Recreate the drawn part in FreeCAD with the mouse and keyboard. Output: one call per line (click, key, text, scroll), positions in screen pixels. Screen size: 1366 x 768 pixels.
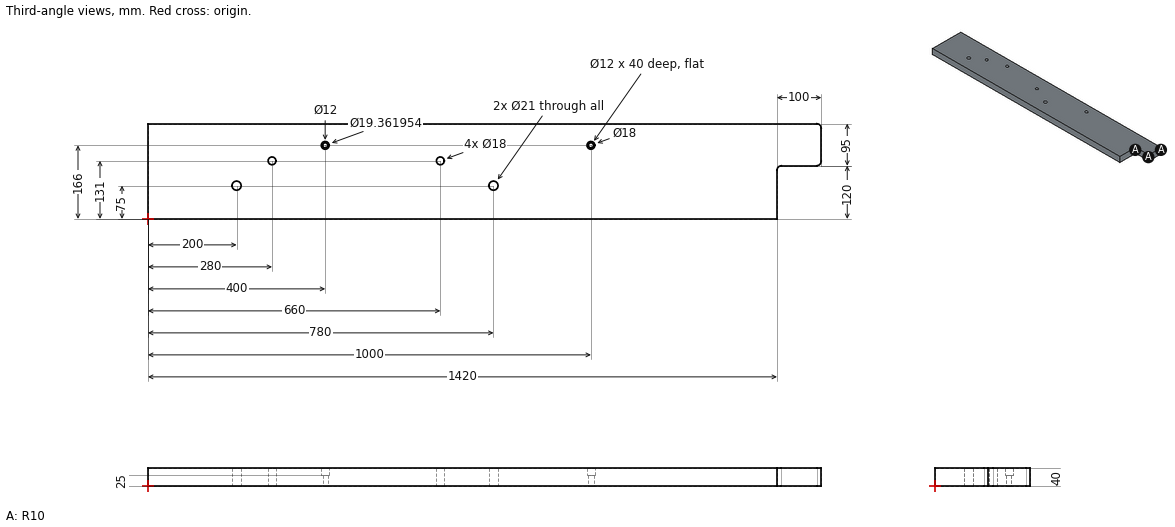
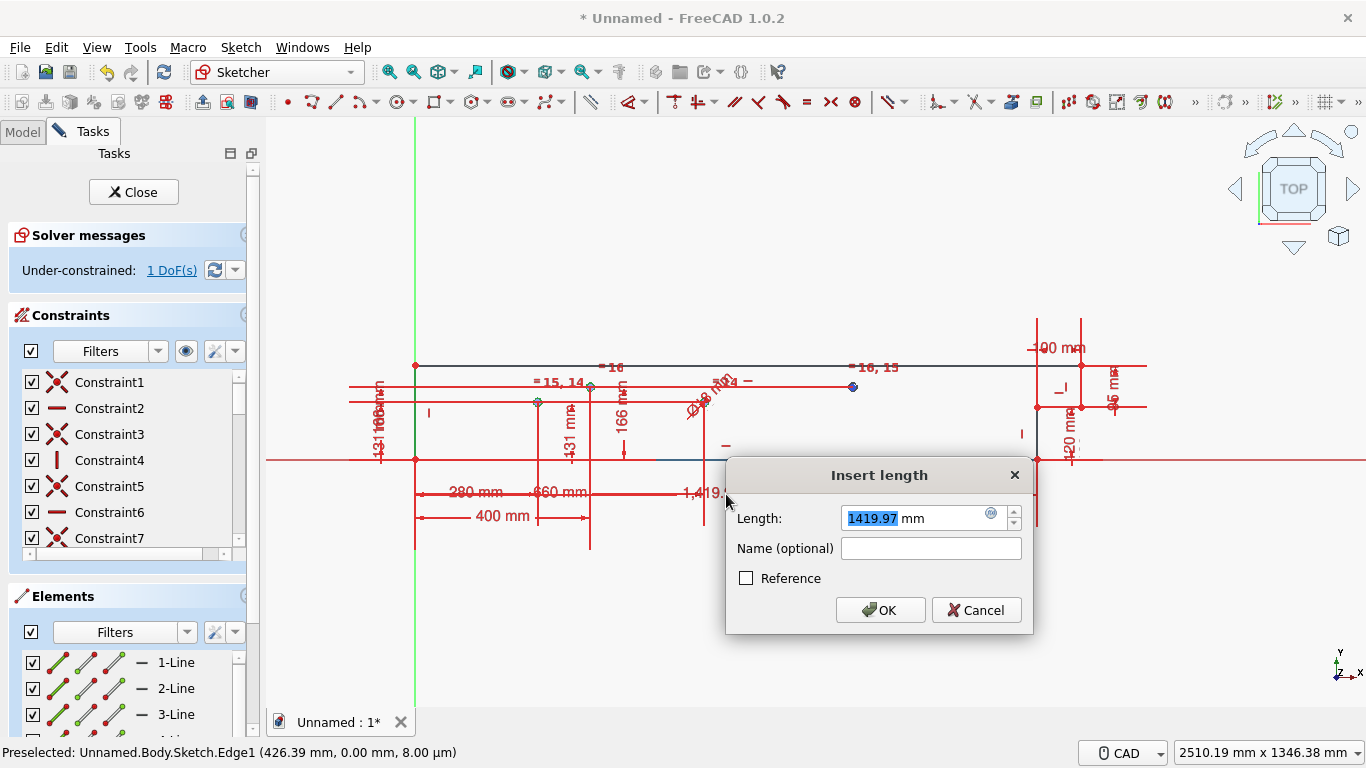
text(1420)
key(Return)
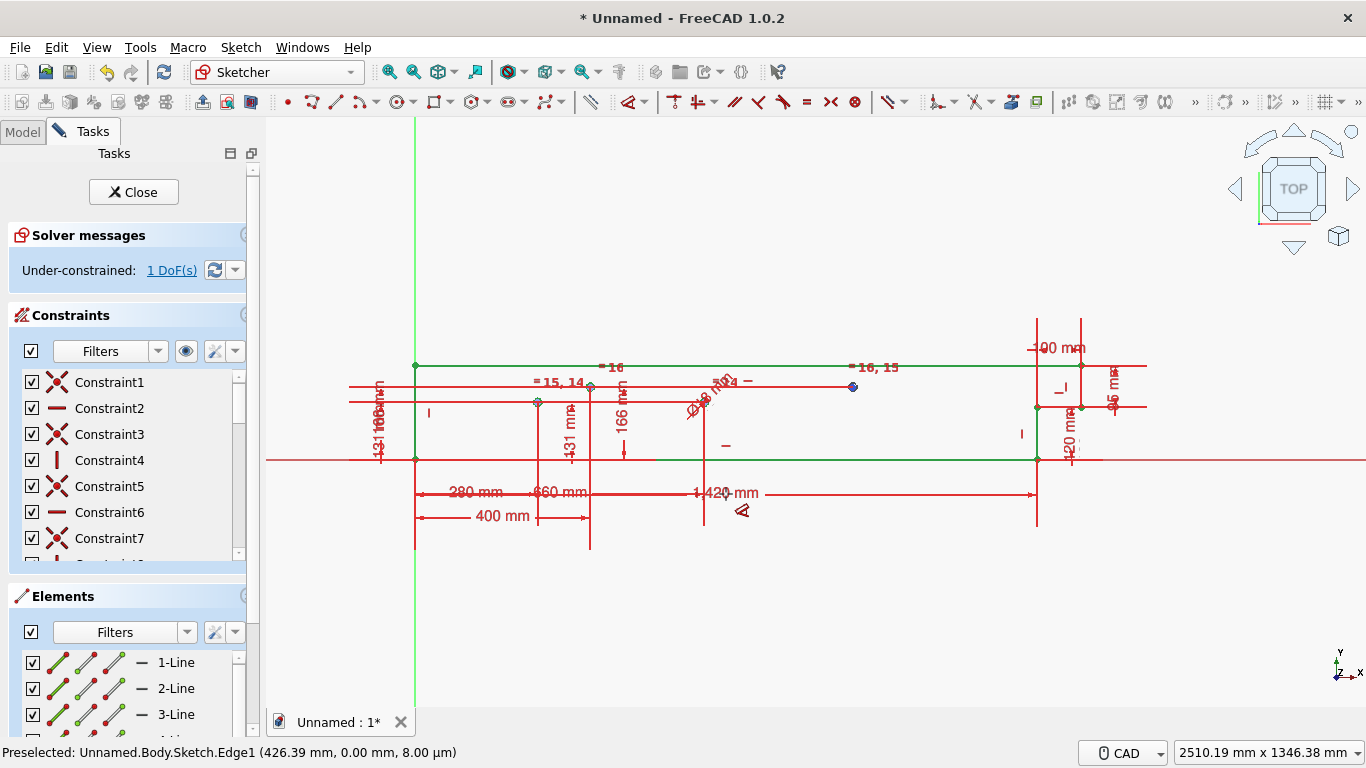
click(853, 387)
click(634, 494)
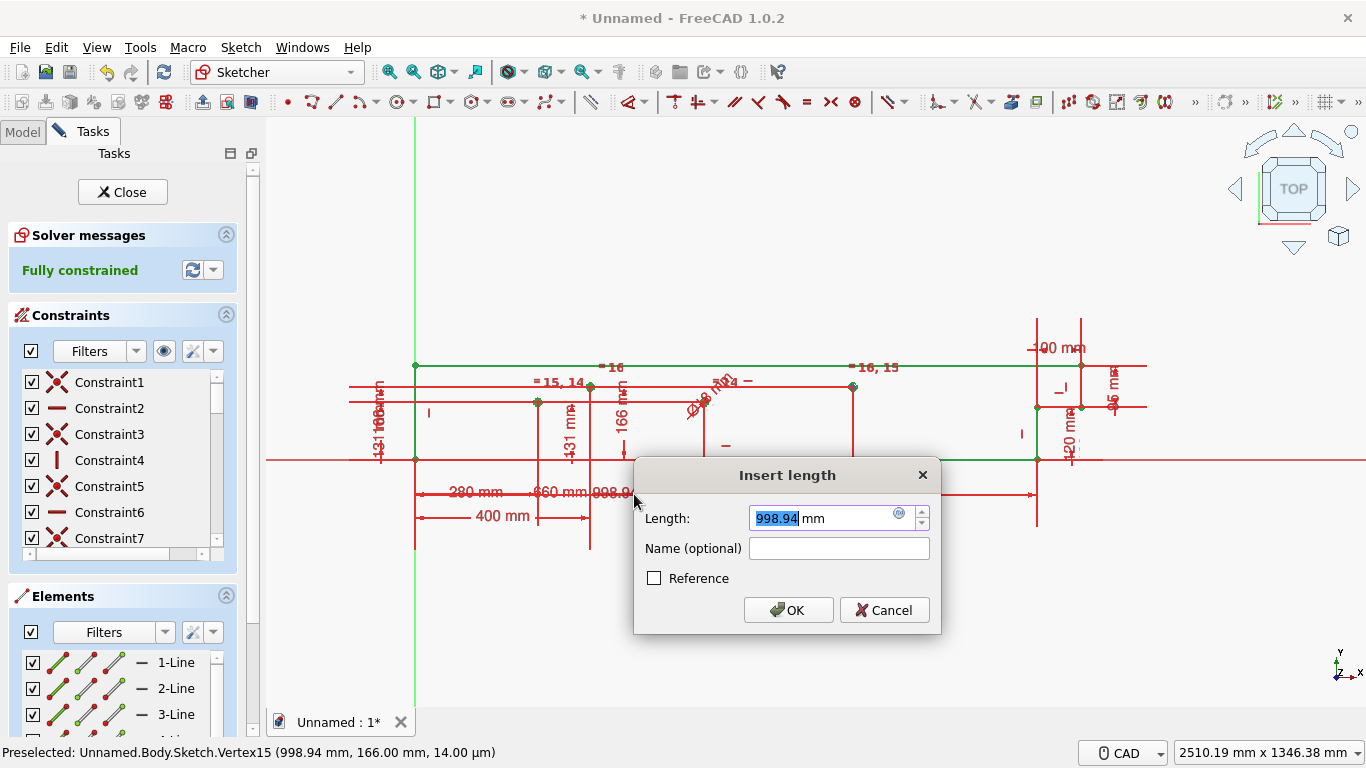
text(1000)
key(Return)
key(Escape)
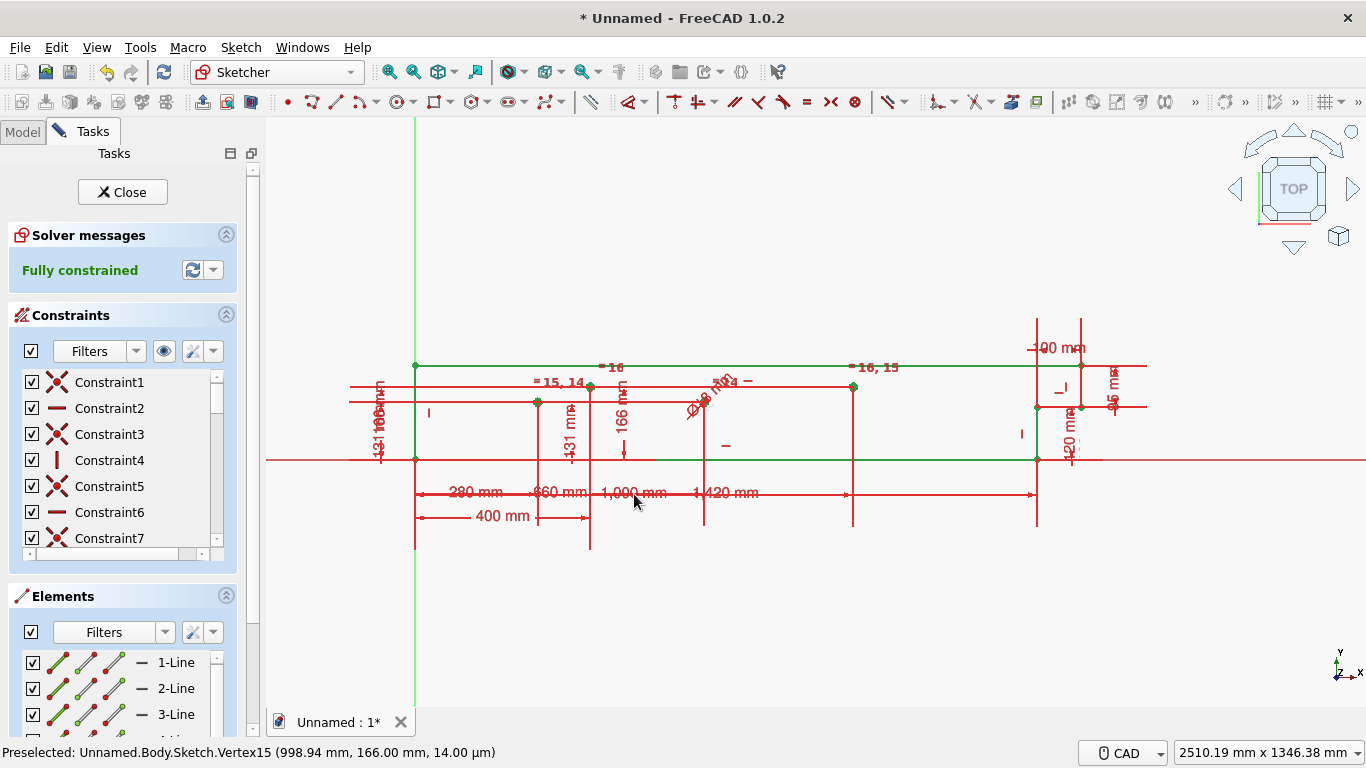
click(123, 192)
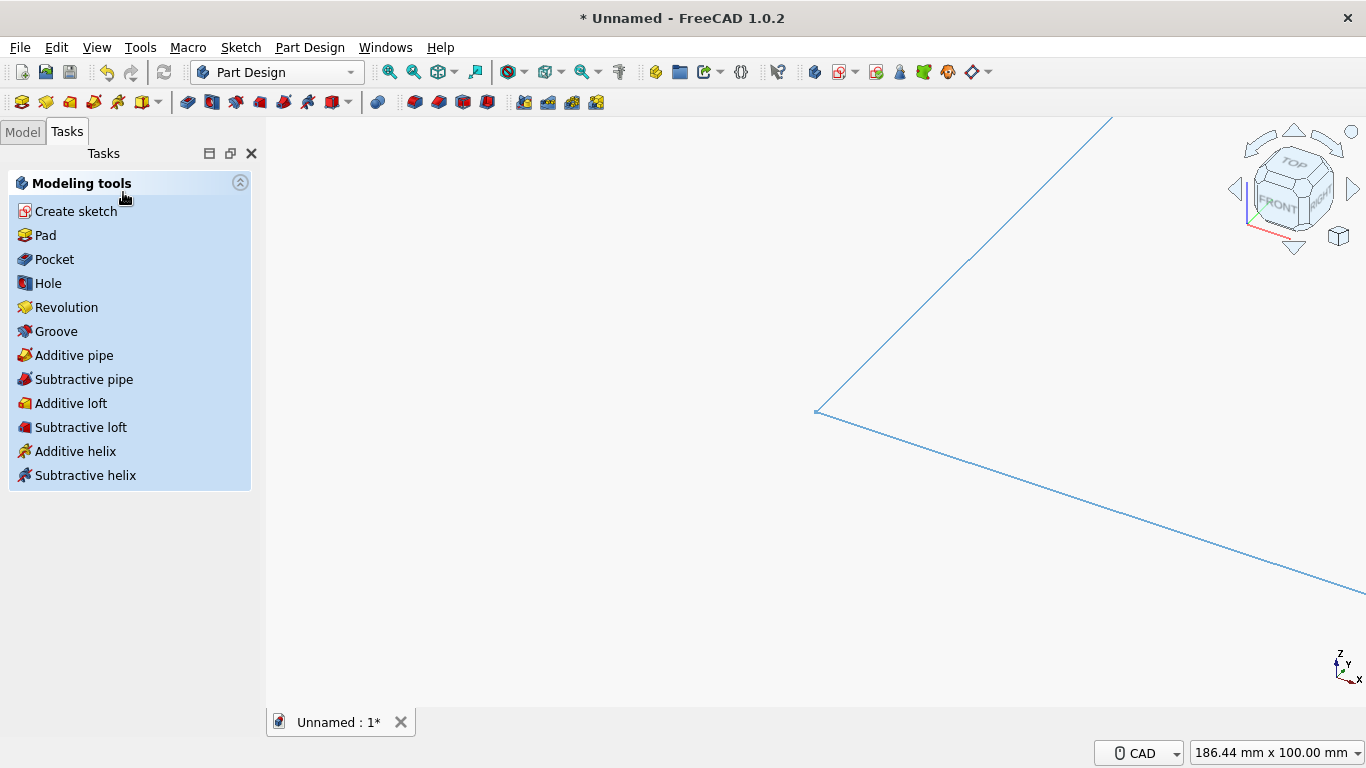
click(22, 102)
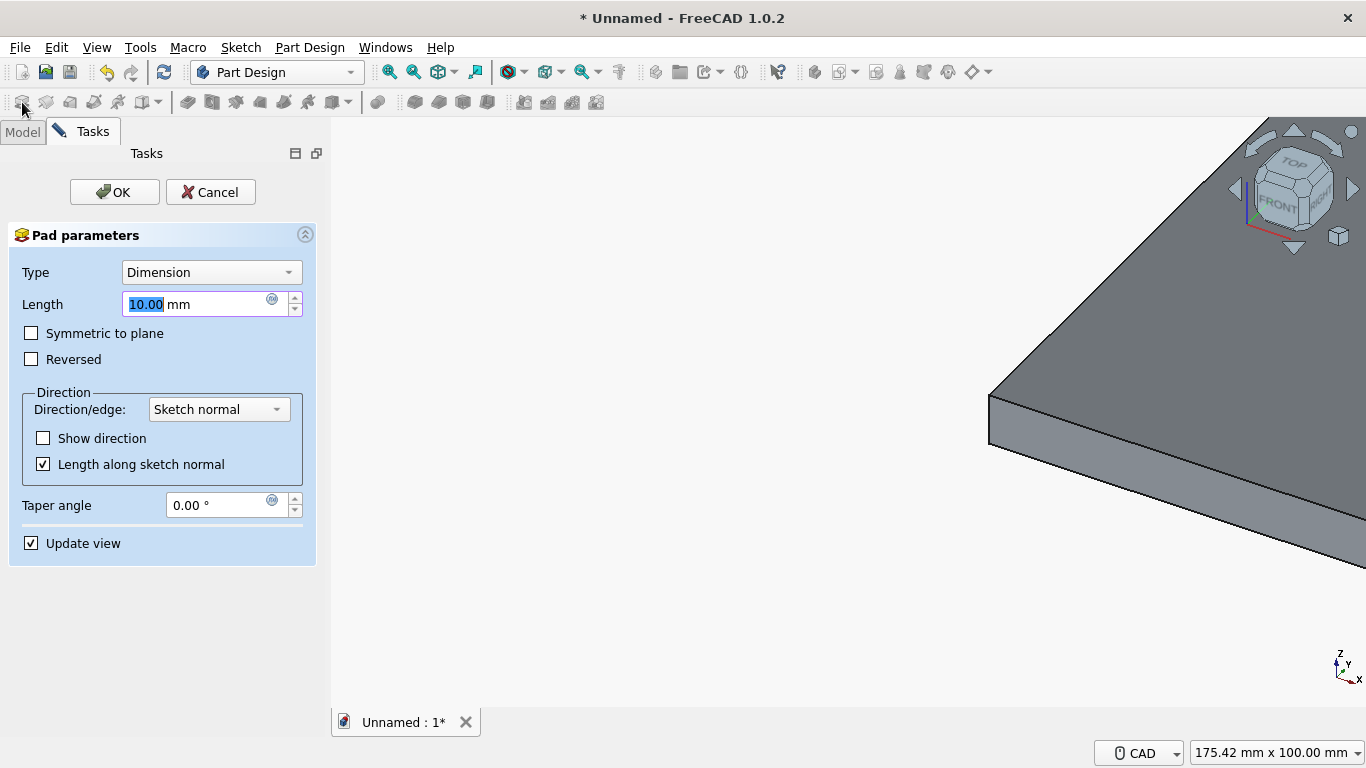
text(40)
key(Tab)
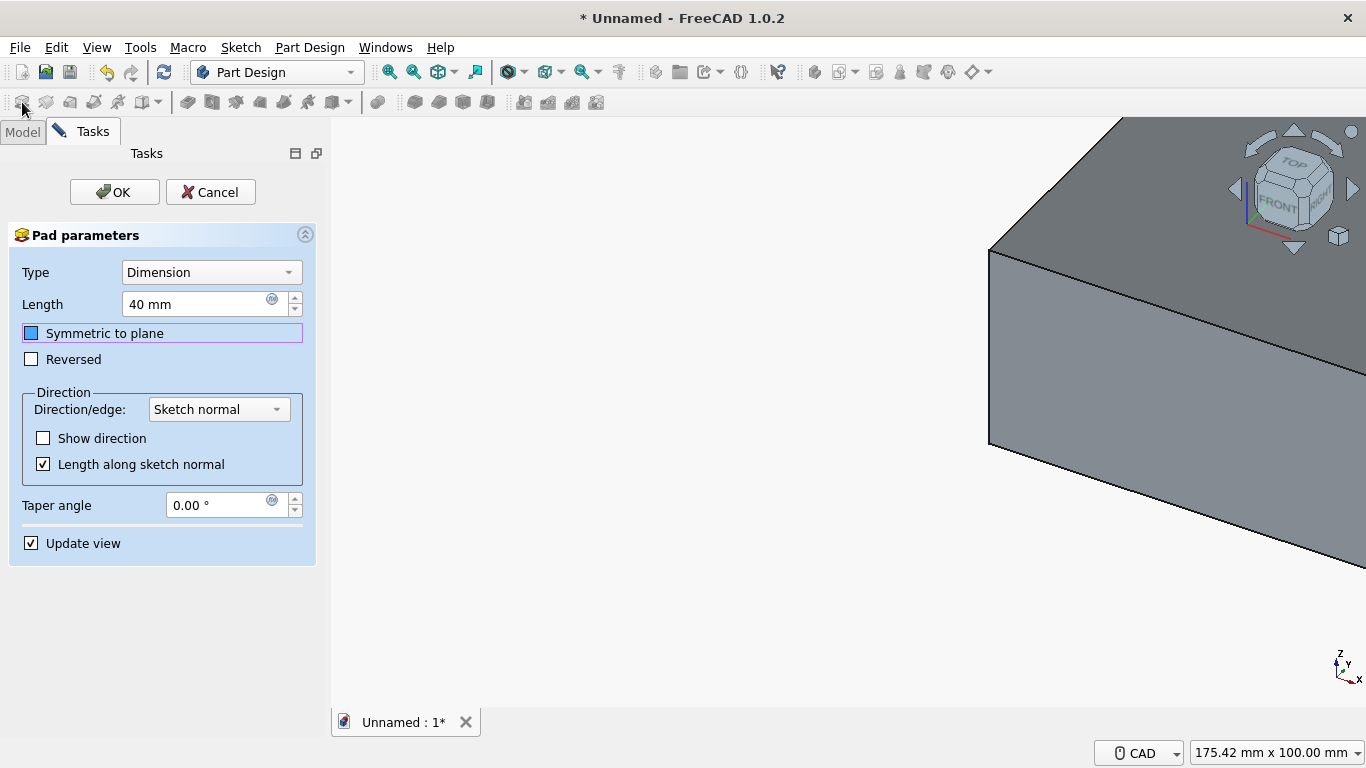
click(115, 192)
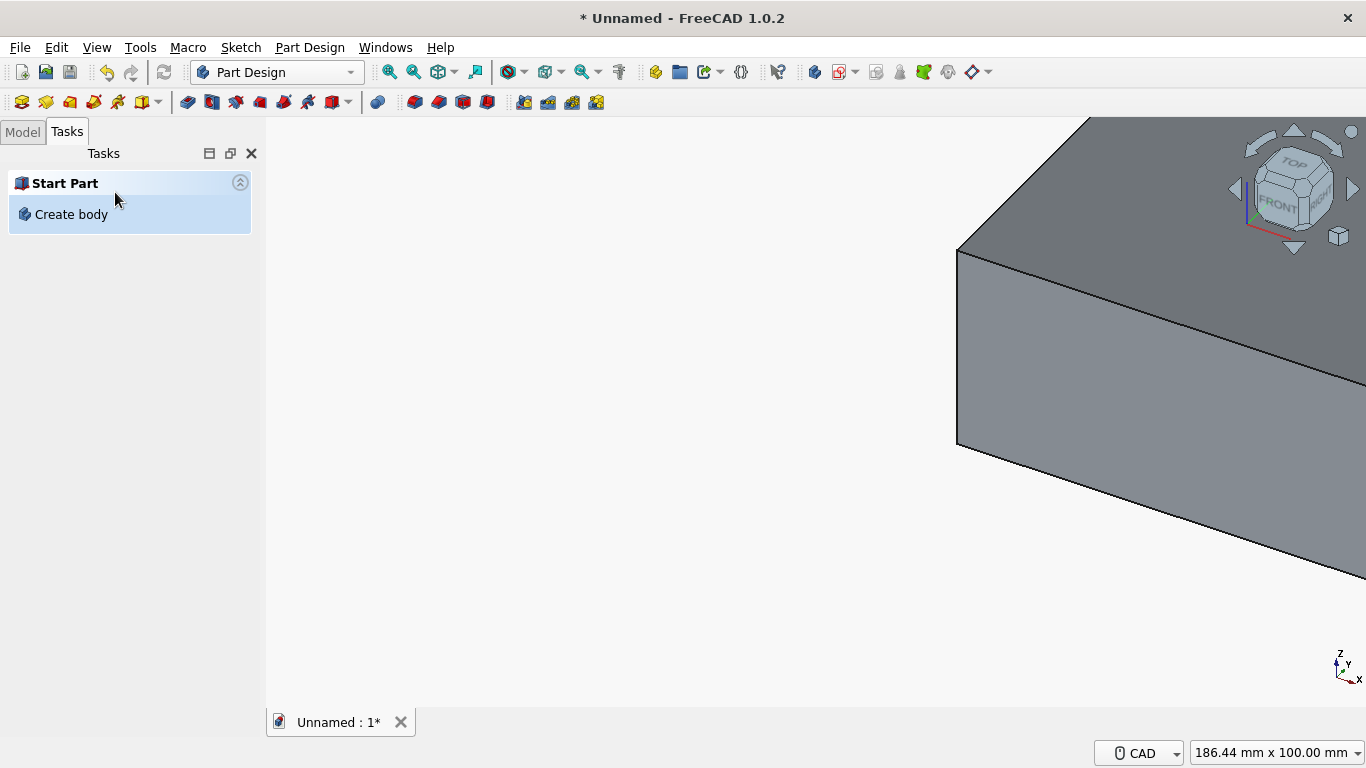
click(390, 72)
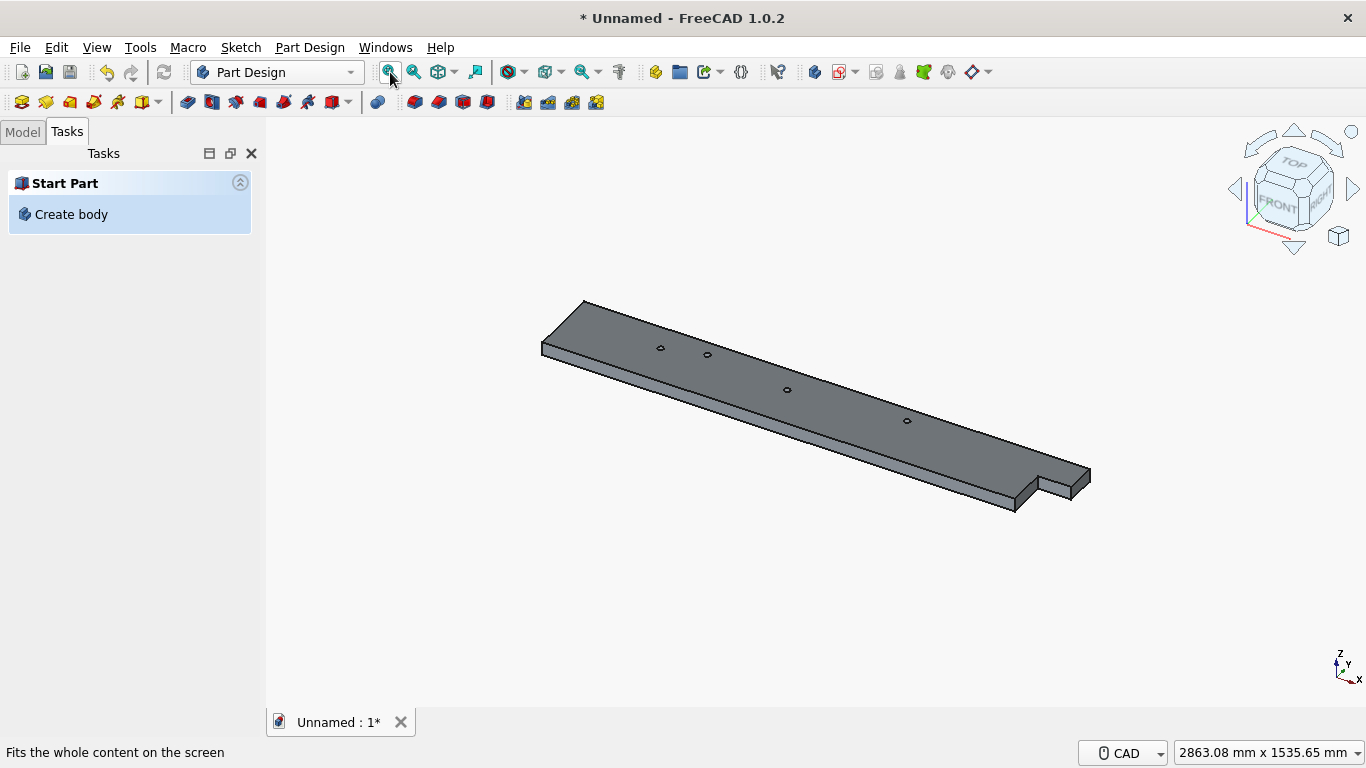
click(960, 453)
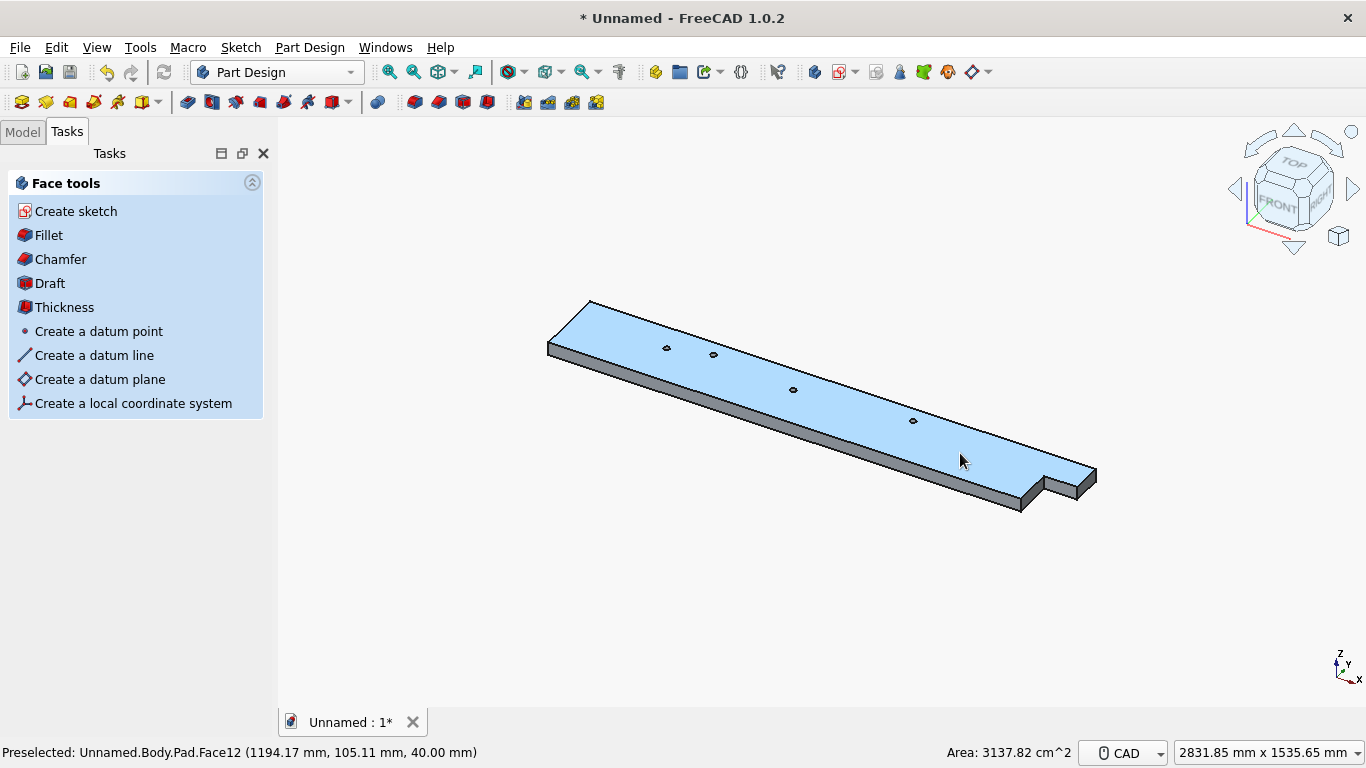
click(840, 72)